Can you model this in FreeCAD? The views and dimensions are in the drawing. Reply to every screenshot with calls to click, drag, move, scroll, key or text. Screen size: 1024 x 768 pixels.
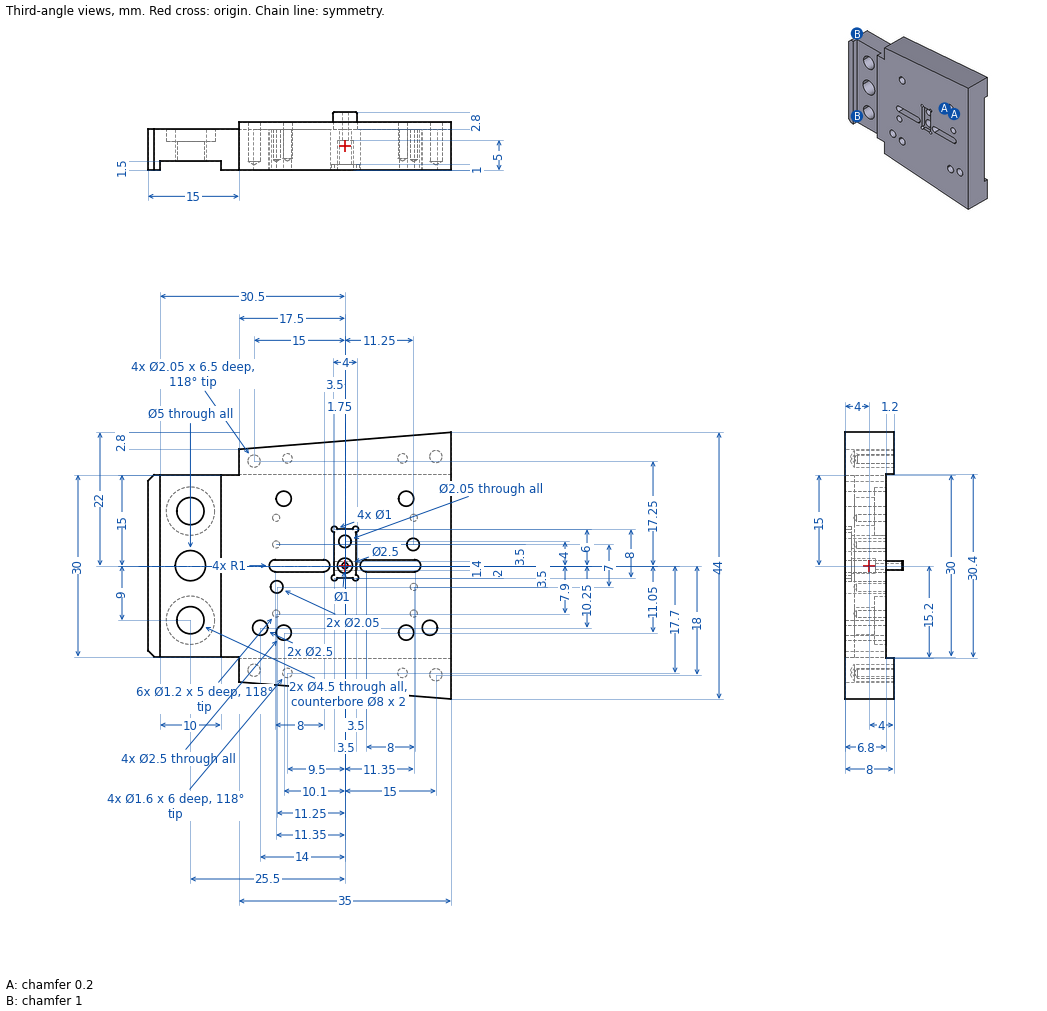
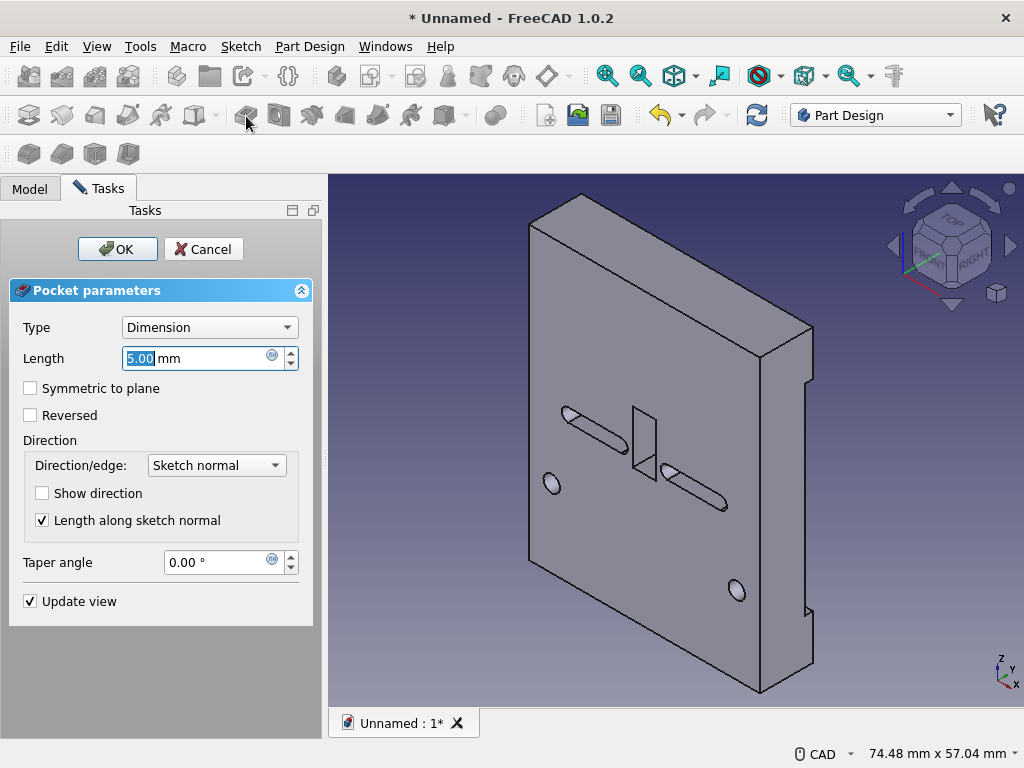
text(1)
key(Tab)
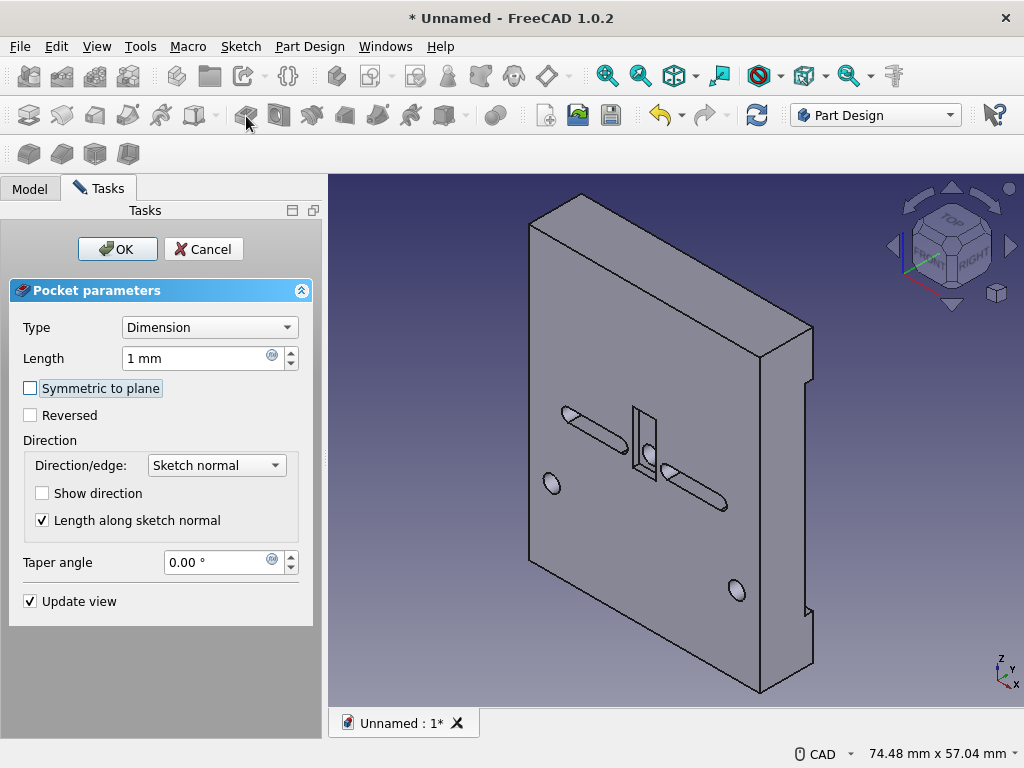
click(118, 249)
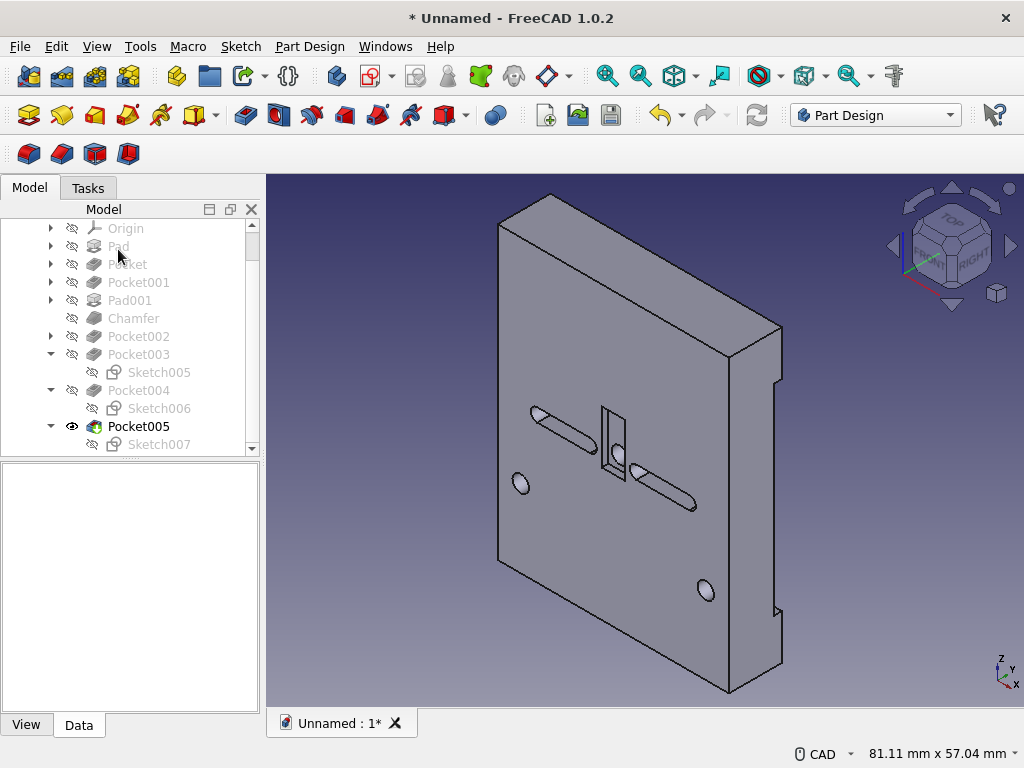
click(613, 554)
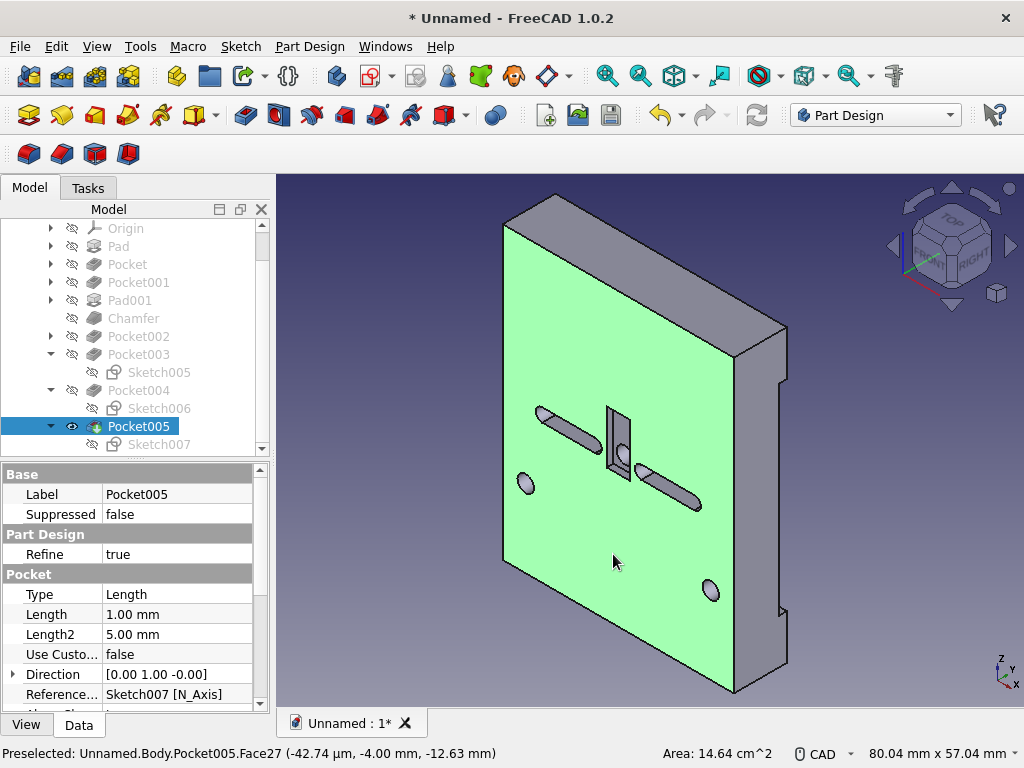
click(370, 76)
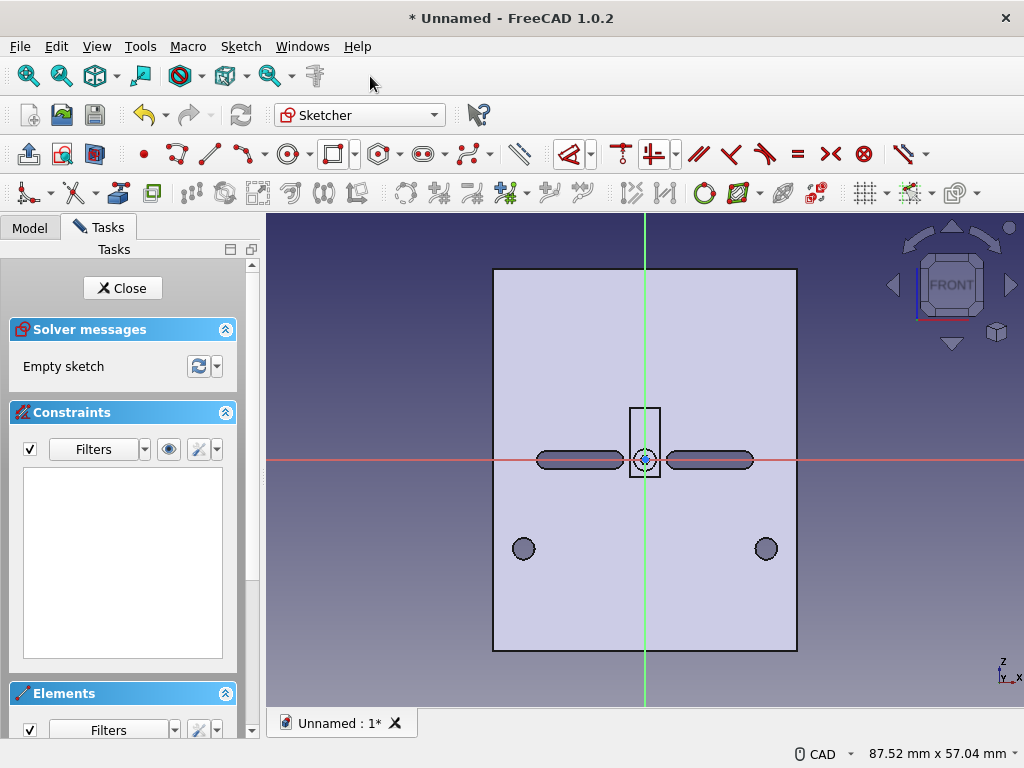
scroll(667, 437, up, 7)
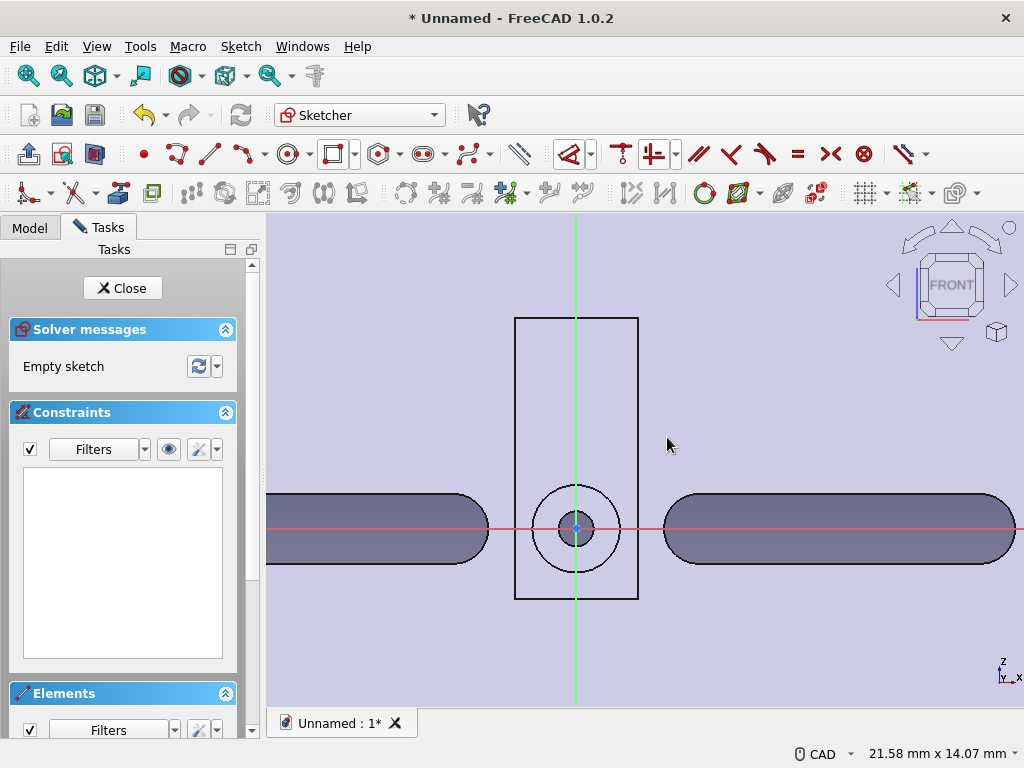
click(288, 154)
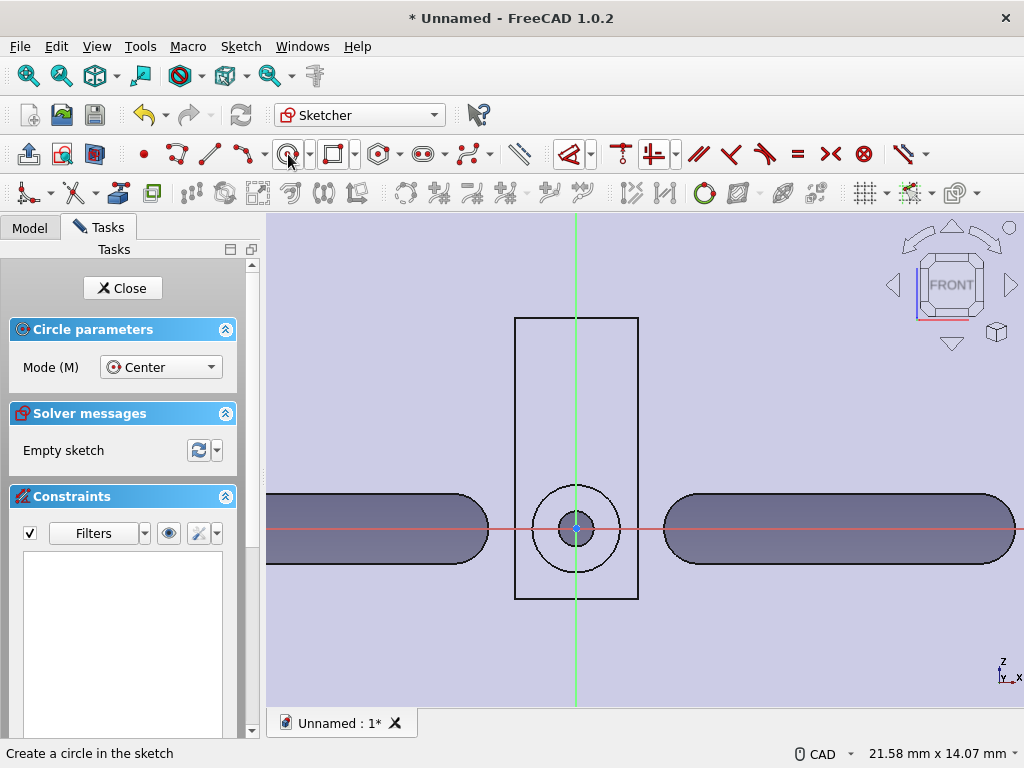
scroll(515, 318, up, 2)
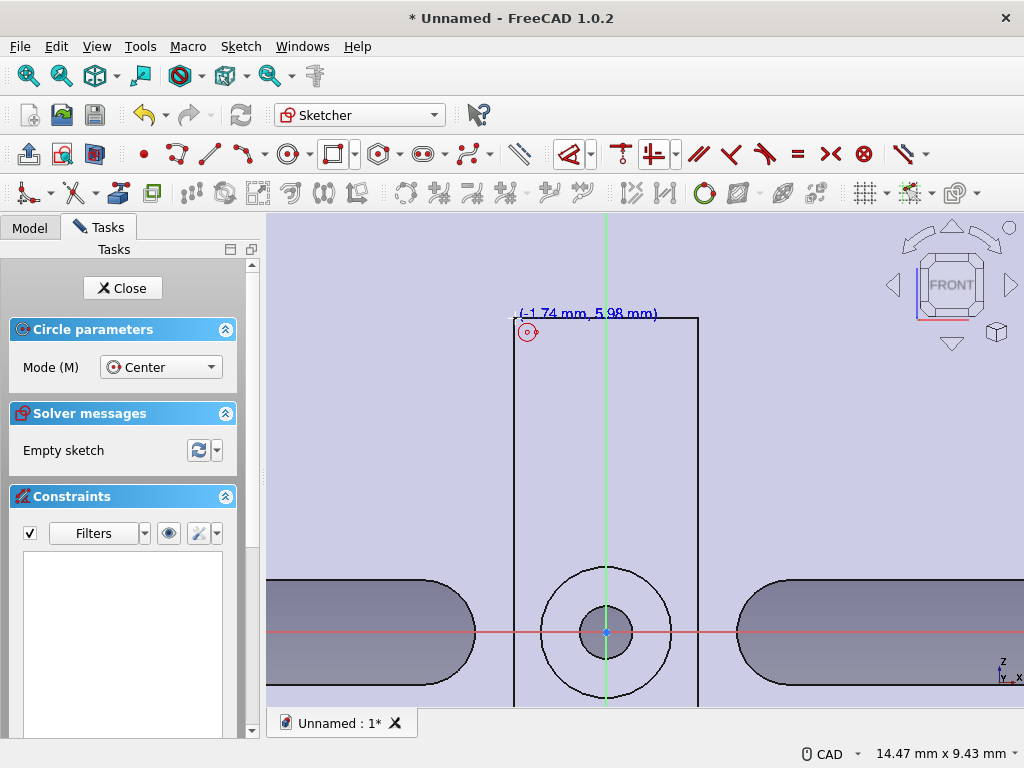
click(514, 318)
move(533, 300)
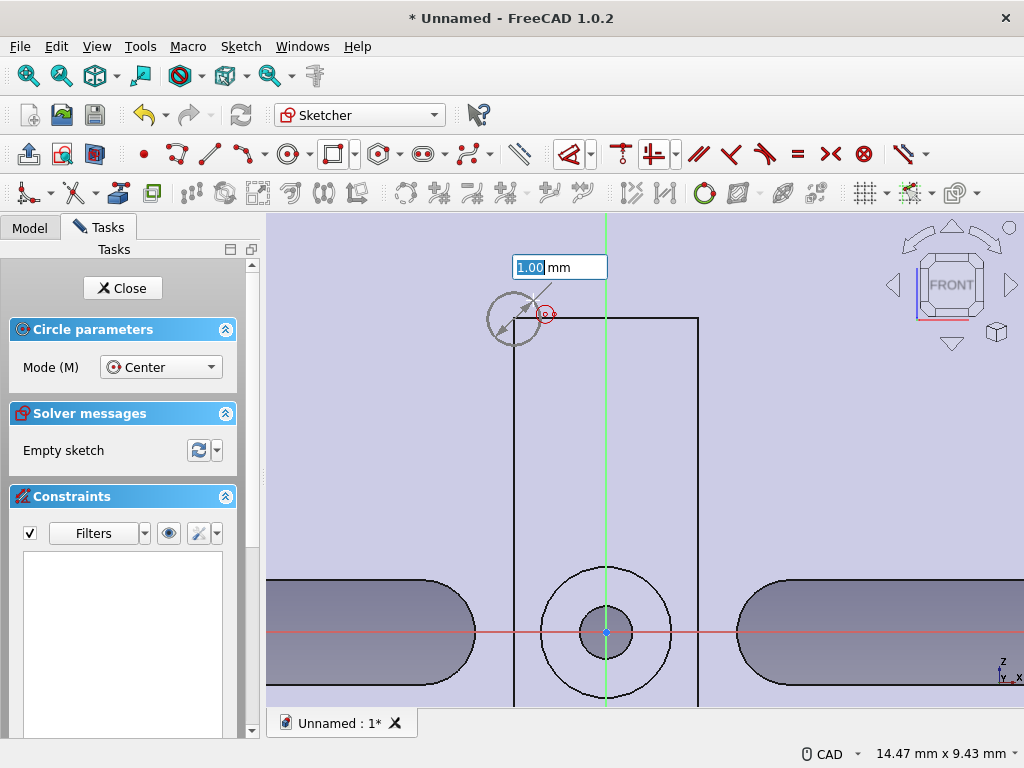
text(1)
key(Return)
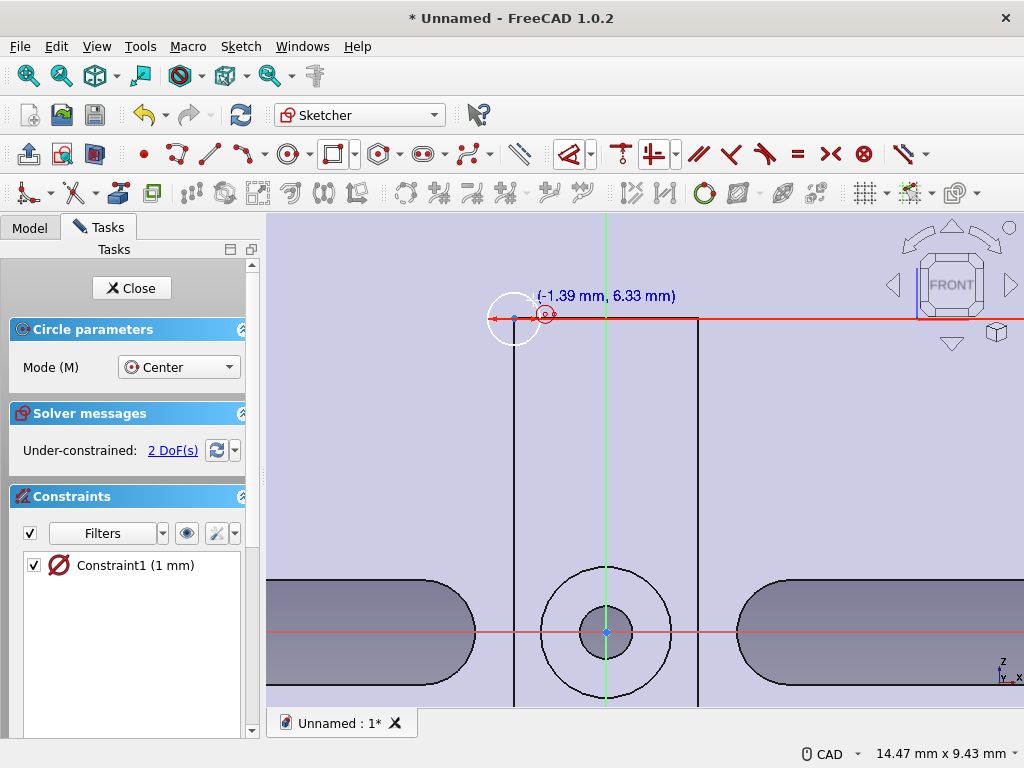
click(698, 318)
move(716, 300)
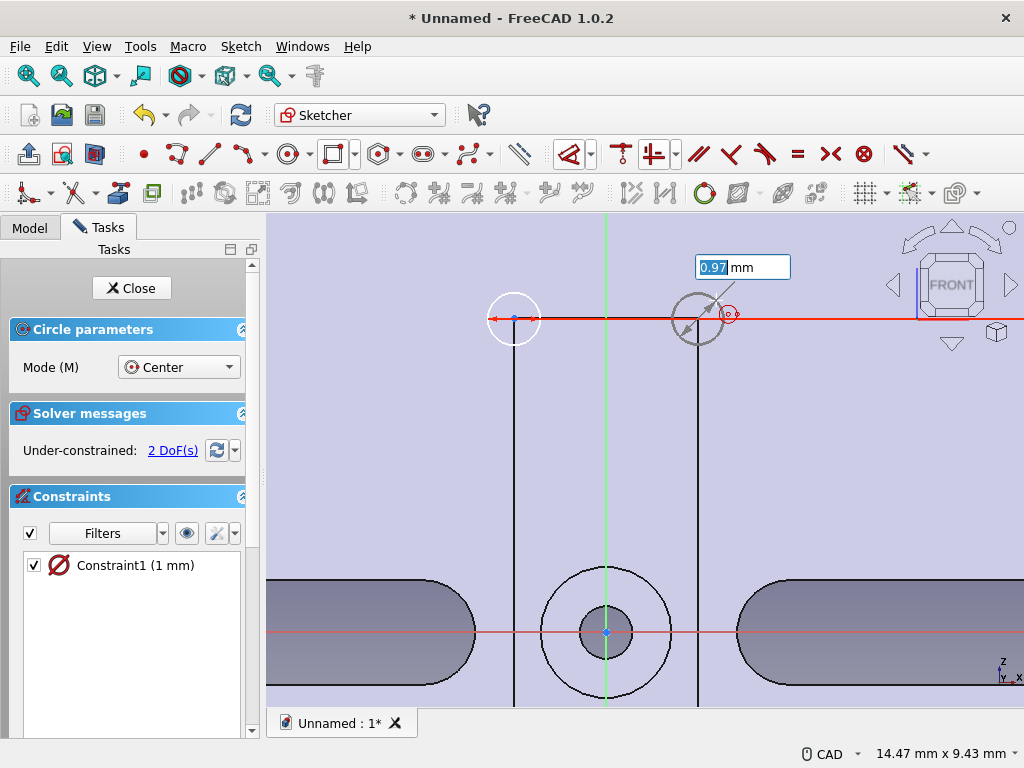
text(1)
key(Return)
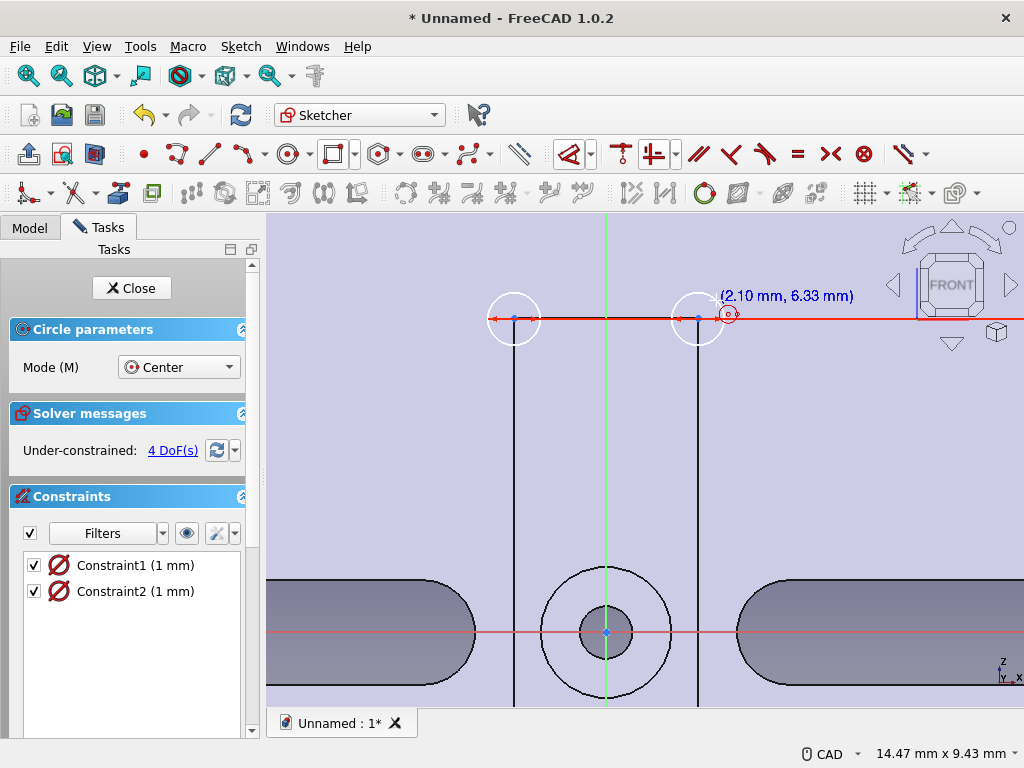
scroll(516, 322, down, 2)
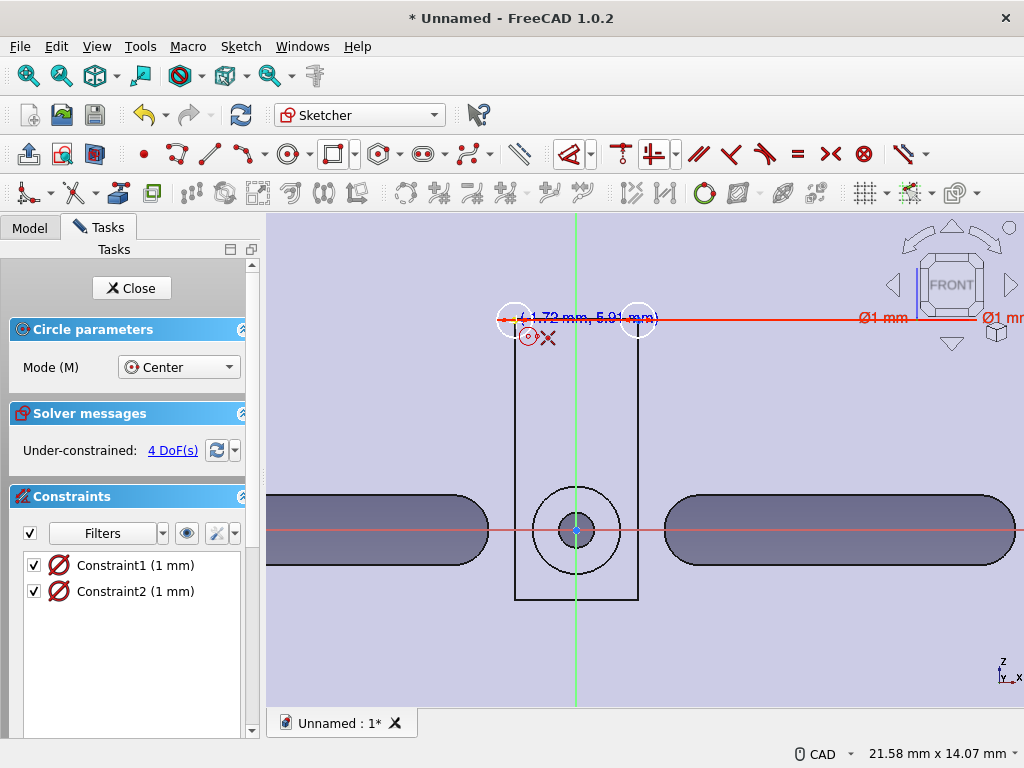
scroll(515, 600, up, 2)